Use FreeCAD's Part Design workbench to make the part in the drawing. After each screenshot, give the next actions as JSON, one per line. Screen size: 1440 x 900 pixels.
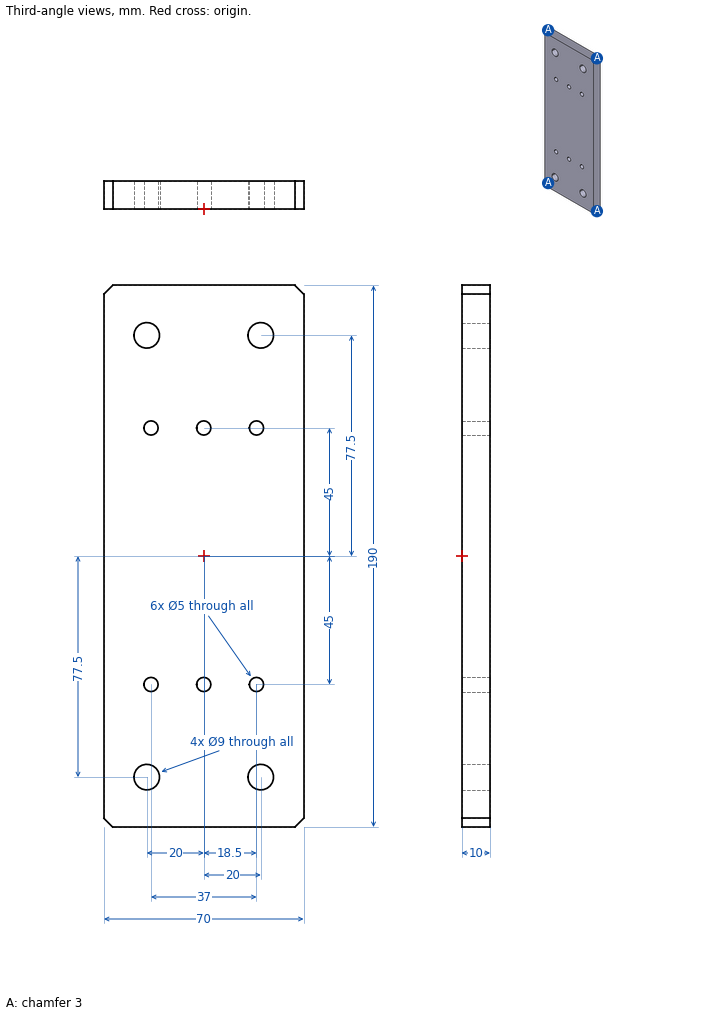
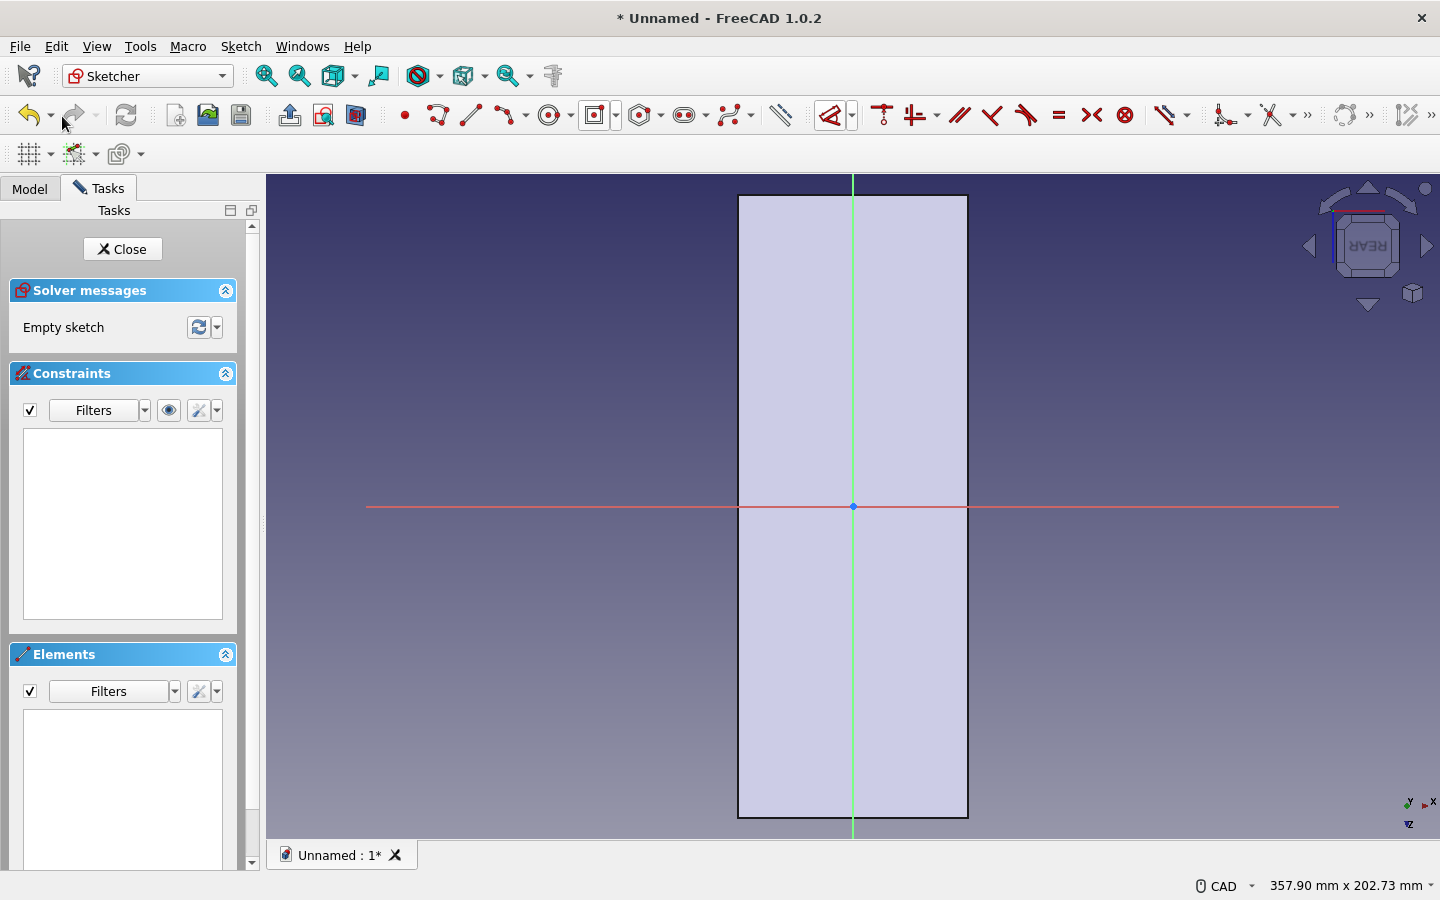
{"action": "scroll", "coordinate": [992, 506], "scroll_direction": "up", "scroll_amount": 2}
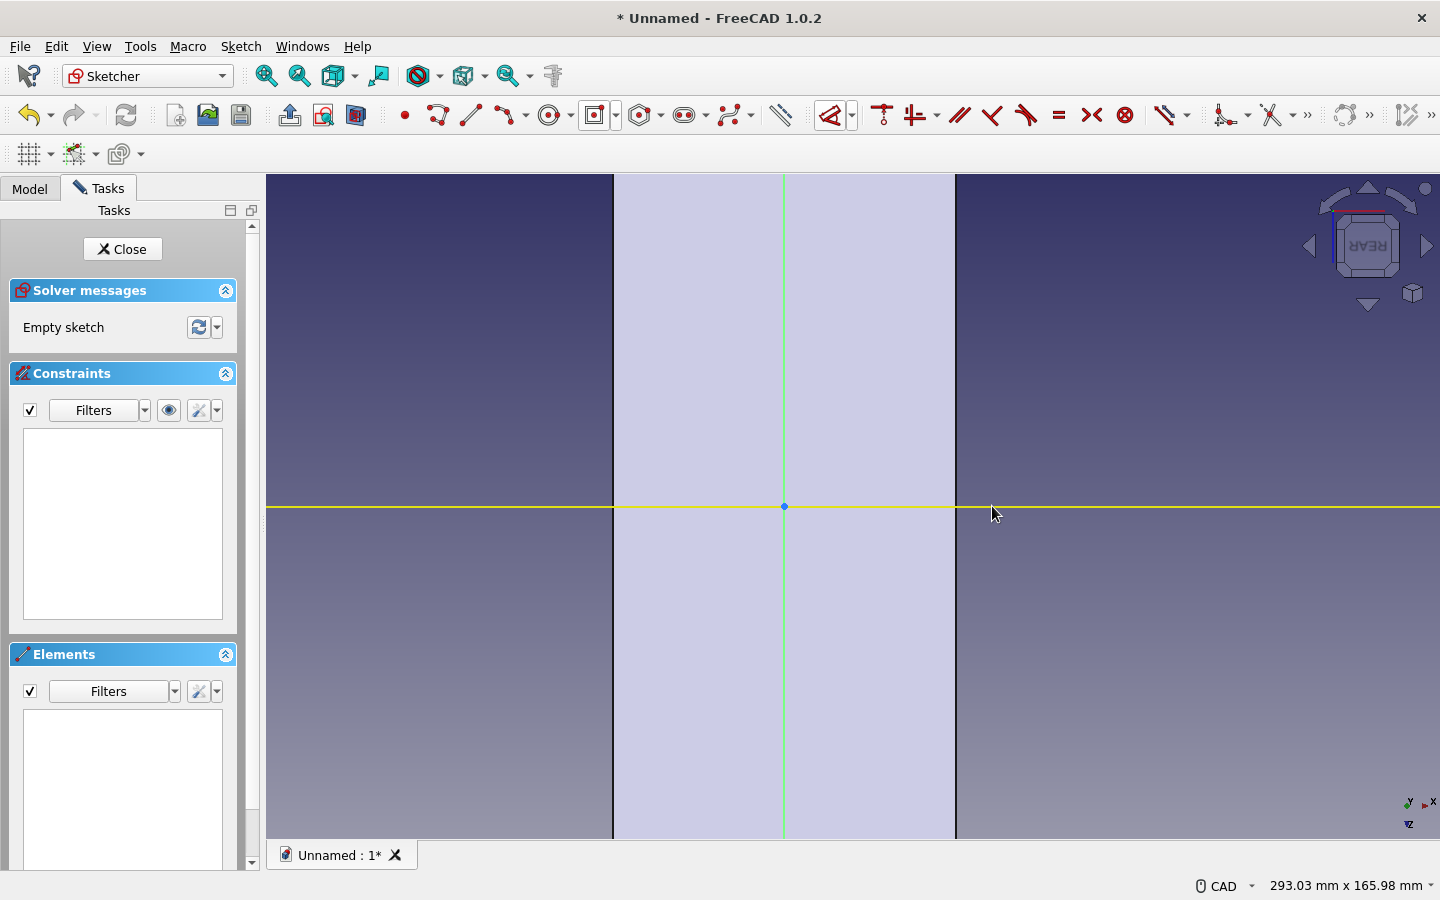
{"action": "left_click", "coordinate": [548, 116]}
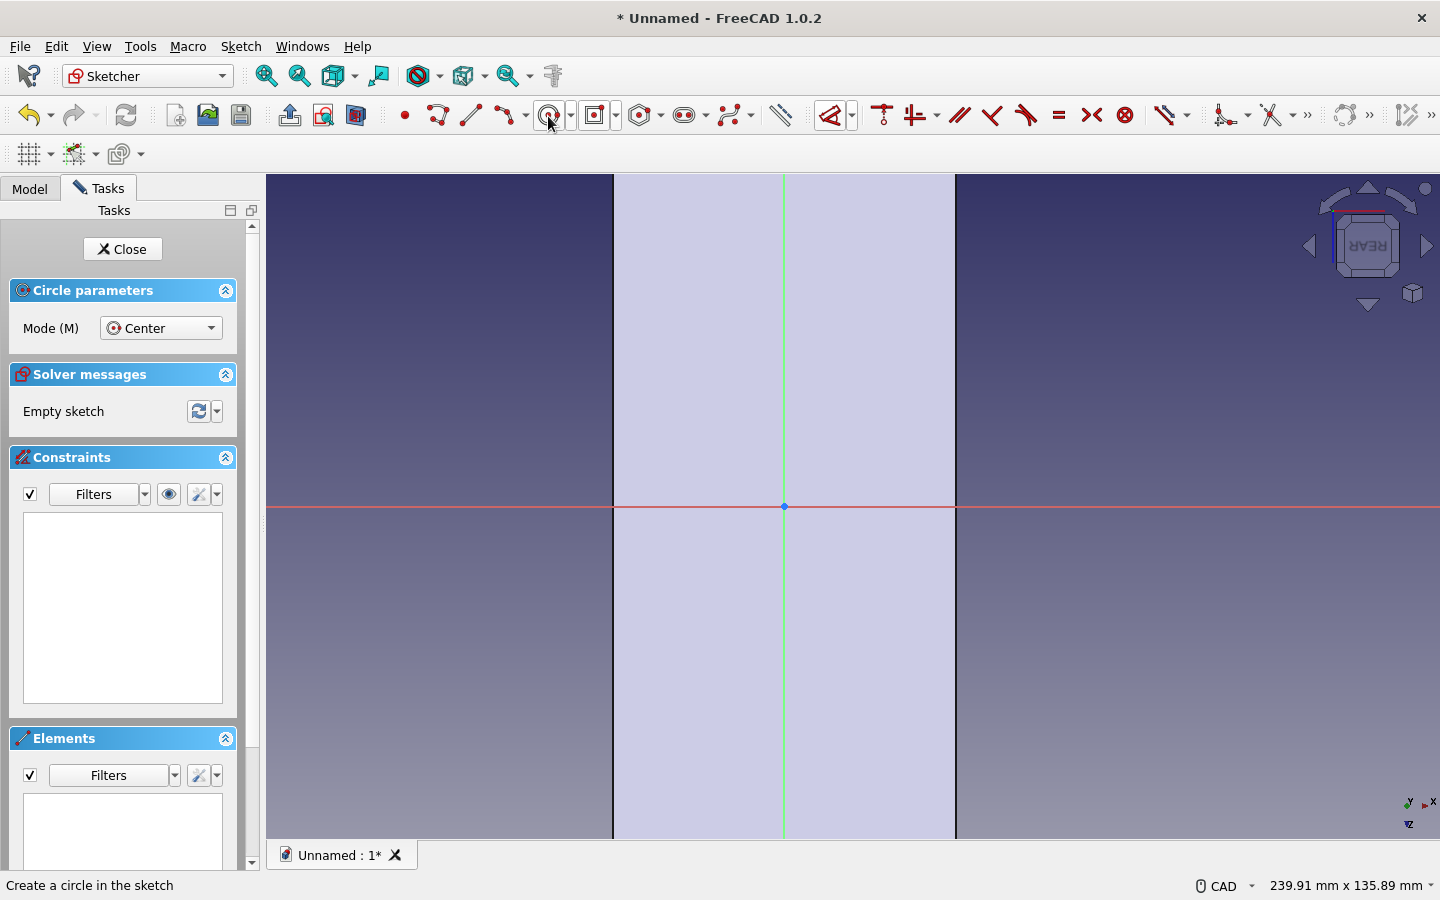
{"action": "scroll", "coordinate": [875, 286], "scroll_direction": "up", "scroll_amount": 4}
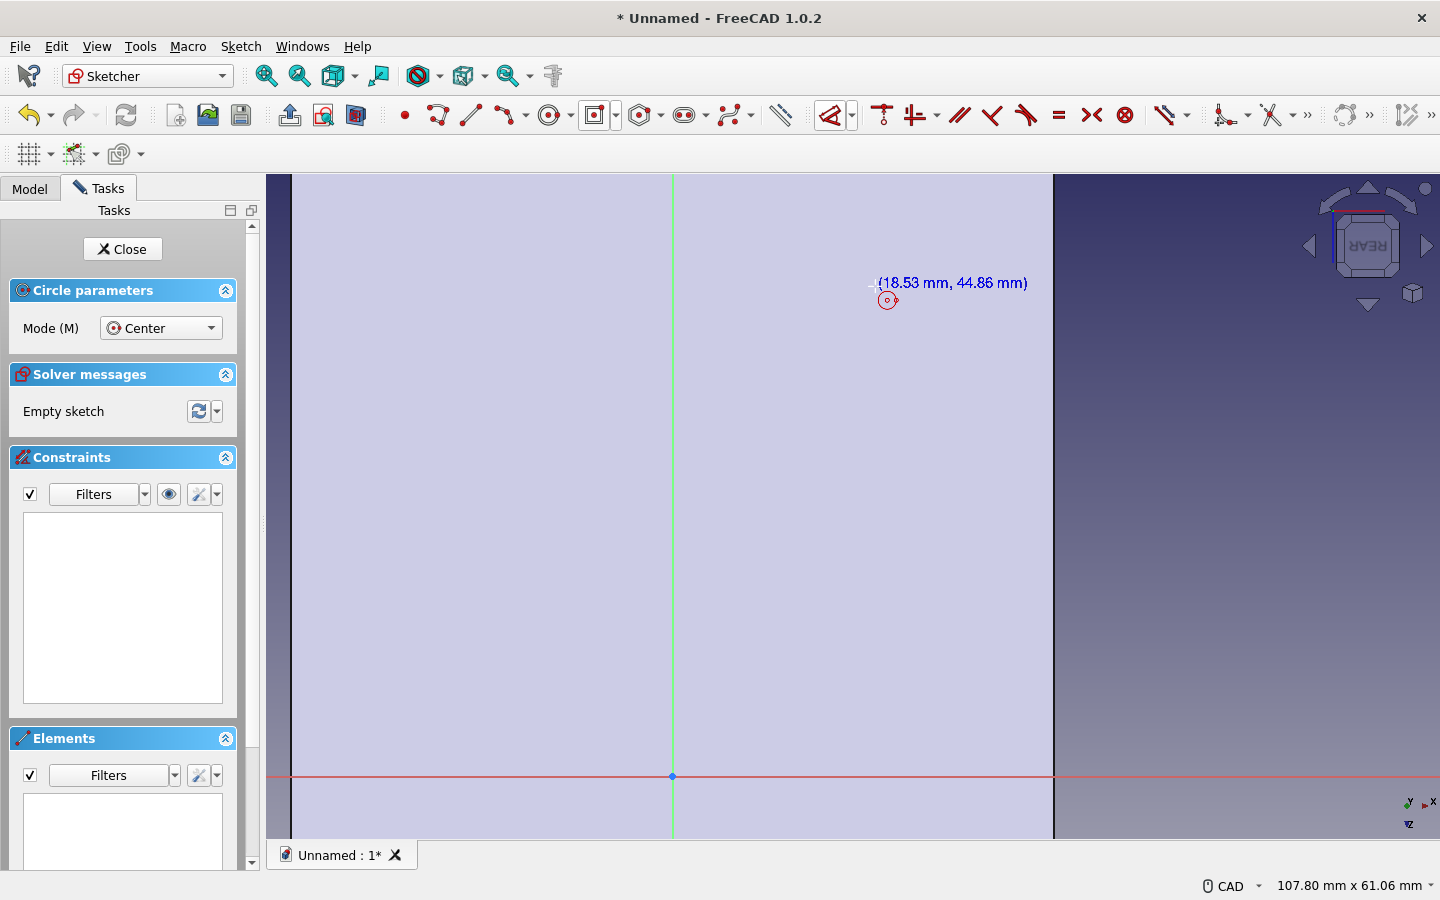
{"action": "left_click", "coordinate": [874, 286]}
{"action": "left_click", "coordinate": [893, 267]}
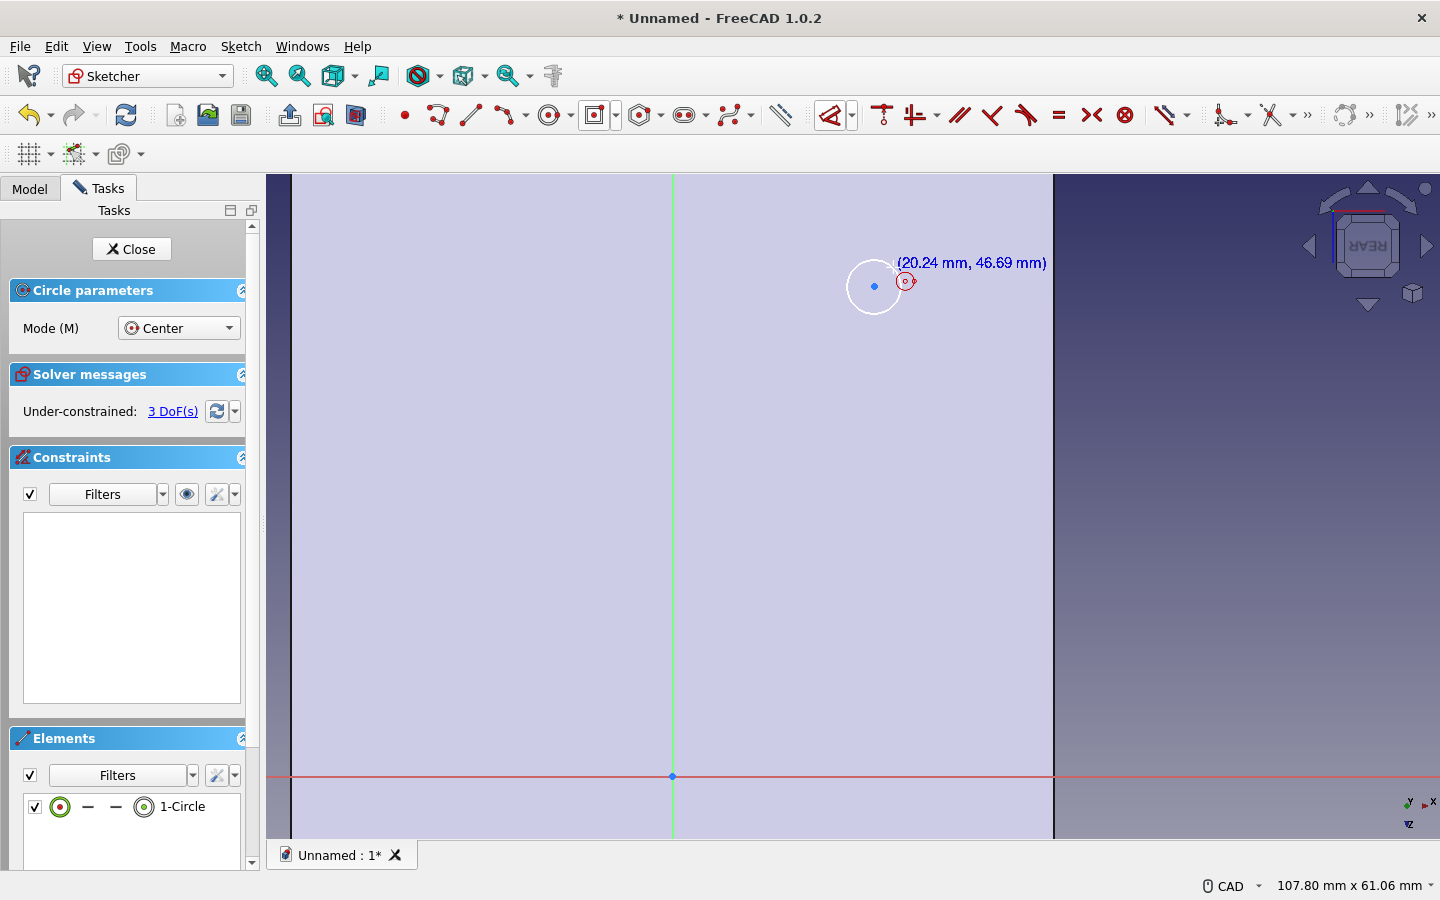
{"action": "left_click", "coordinate": [471, 286]}
{"action": "left_click", "coordinate": [490, 267]}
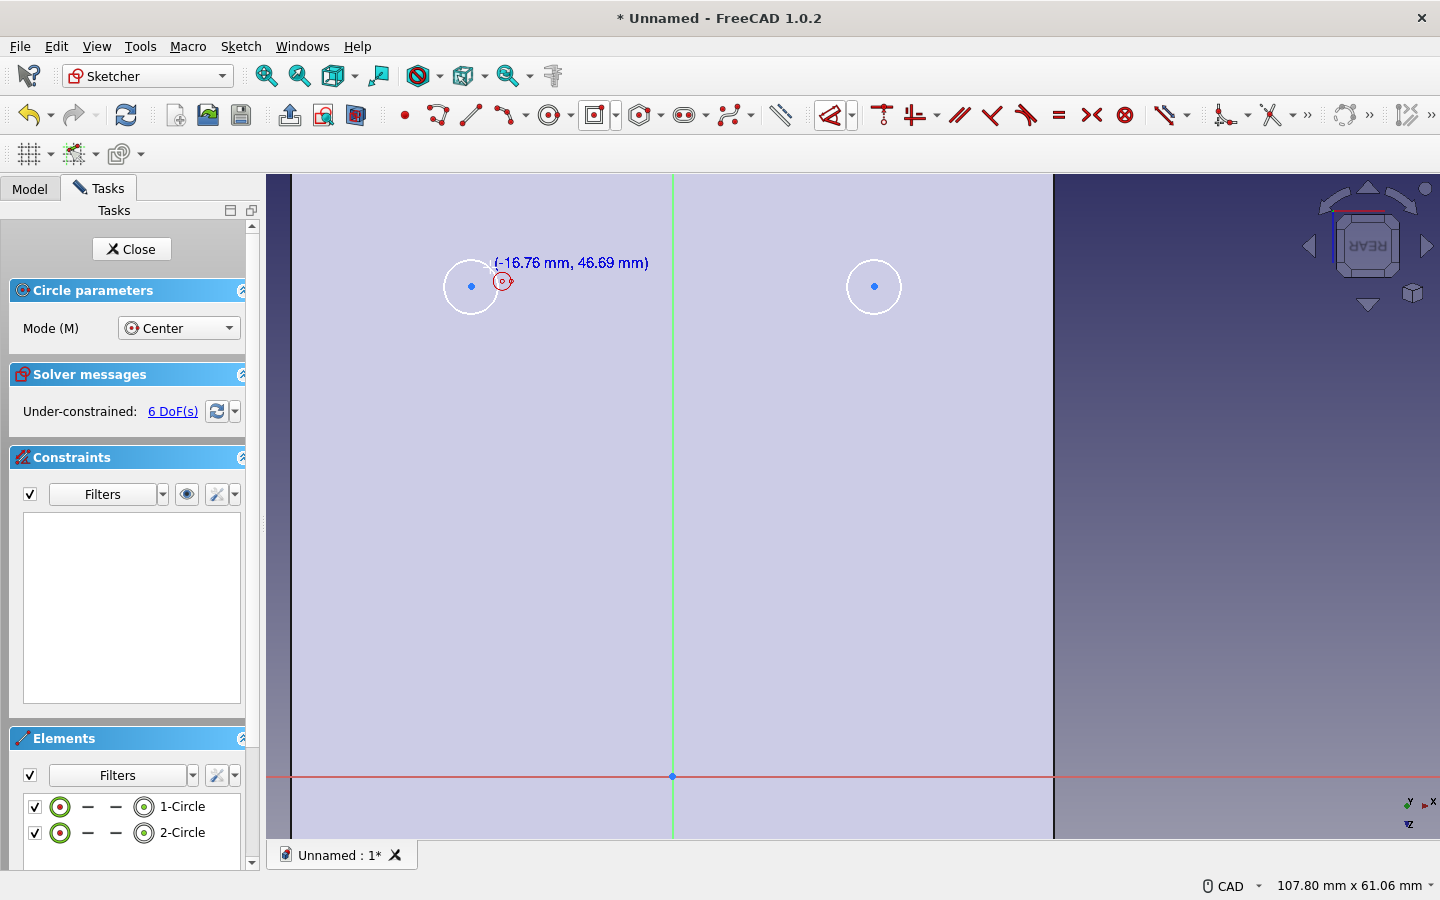
{"action": "left_click", "coordinate": [673, 286]}
{"action": "left_click", "coordinate": [692, 267]}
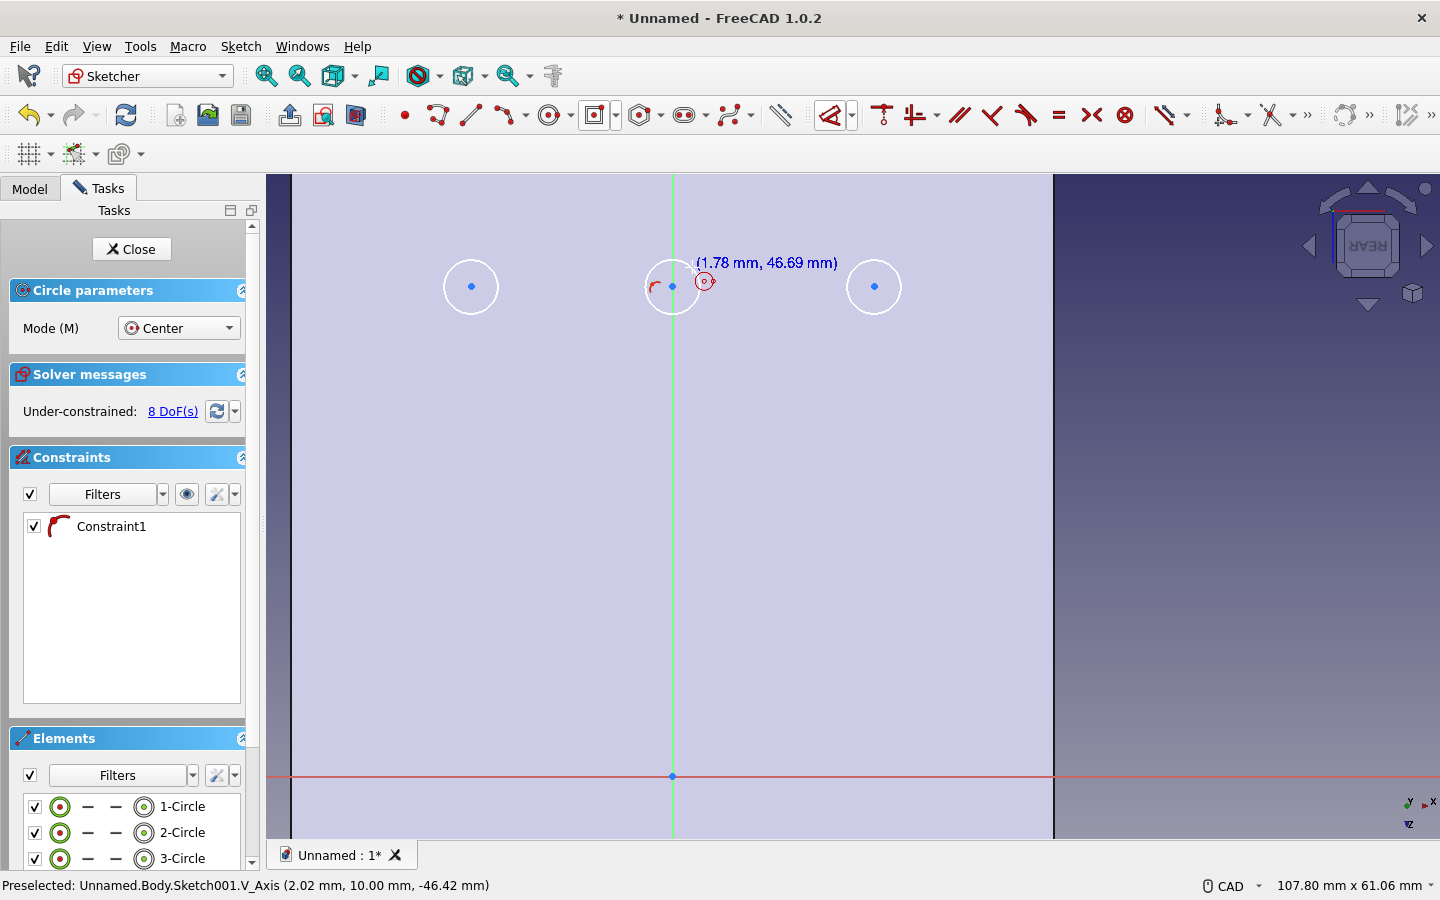
{"action": "scroll", "coordinate": [876, 286], "scroll_direction": "down", "scroll_amount": 4}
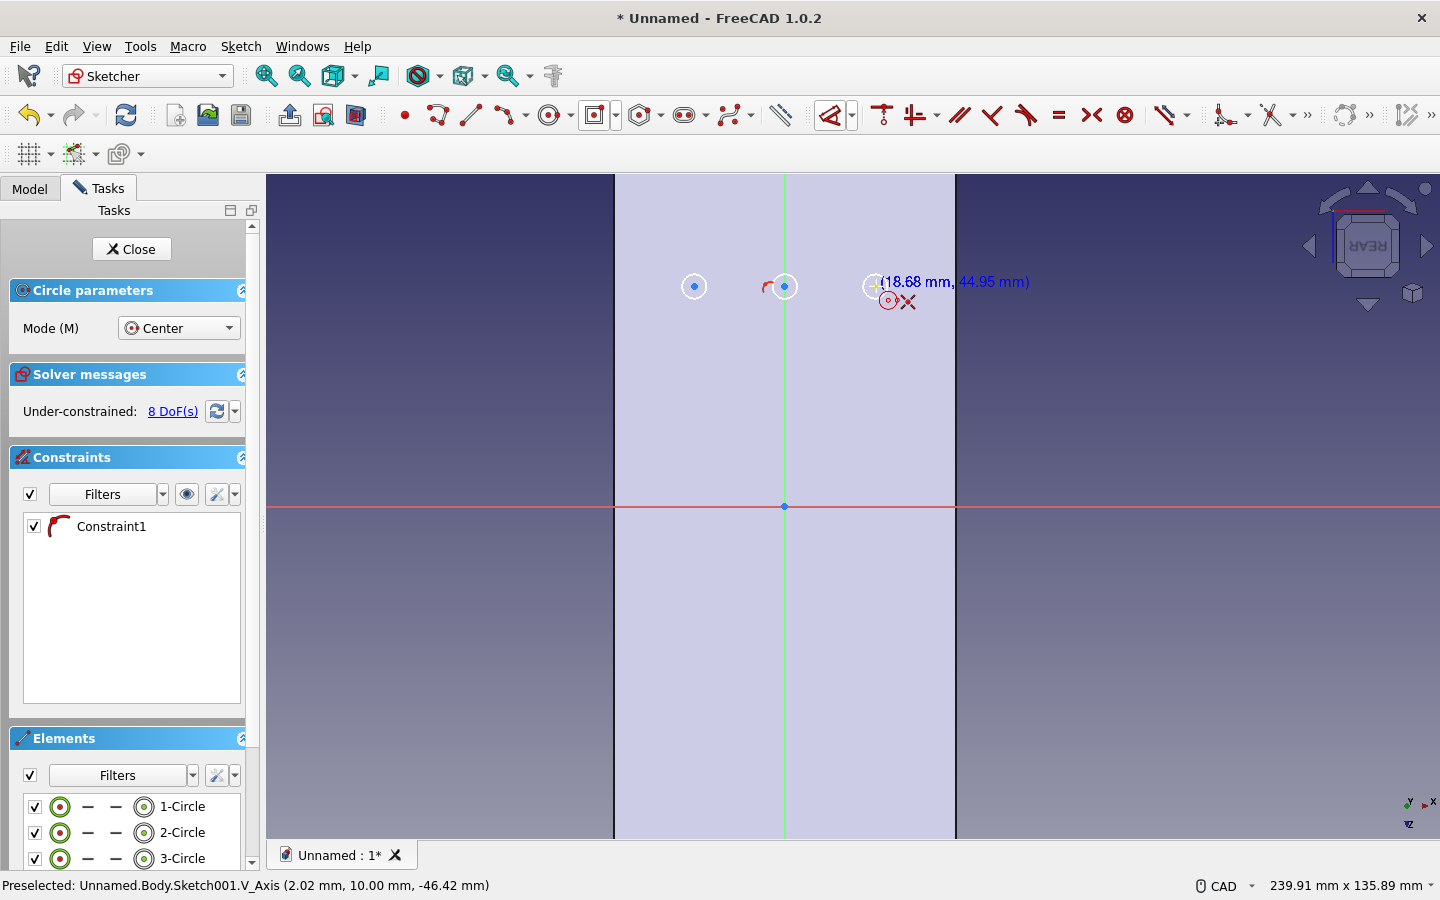
{"action": "scroll", "coordinate": [785, 727], "scroll_direction": "up", "scroll_amount": 4}